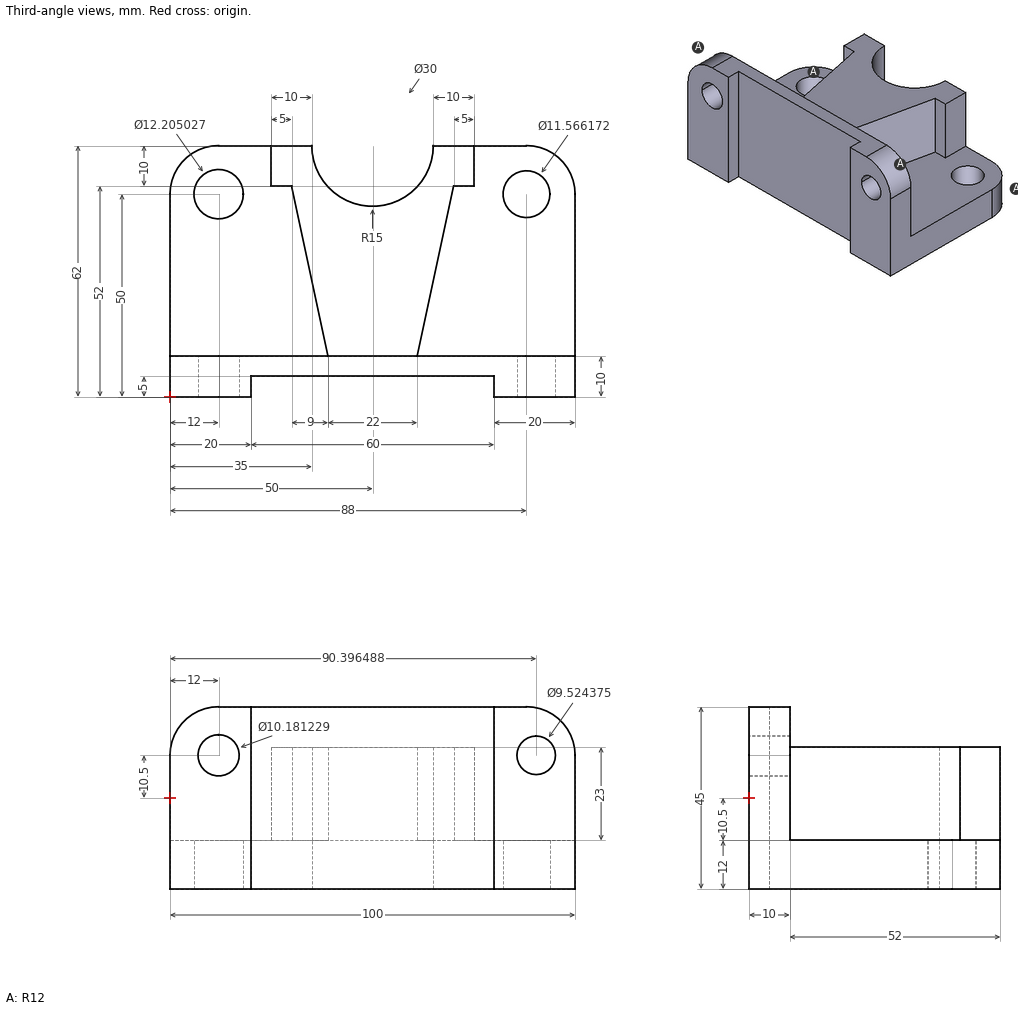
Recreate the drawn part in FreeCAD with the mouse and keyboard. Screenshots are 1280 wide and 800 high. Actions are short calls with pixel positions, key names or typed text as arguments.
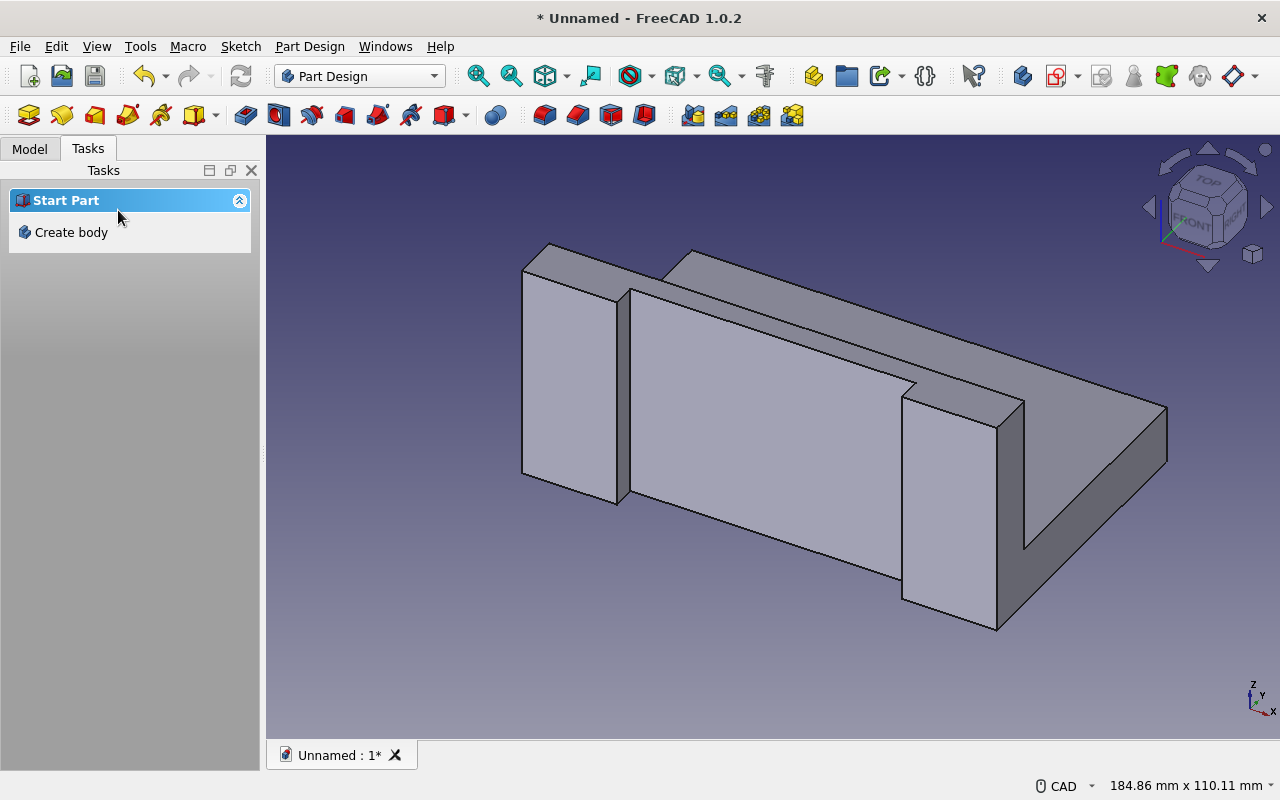
key(v)
key(f)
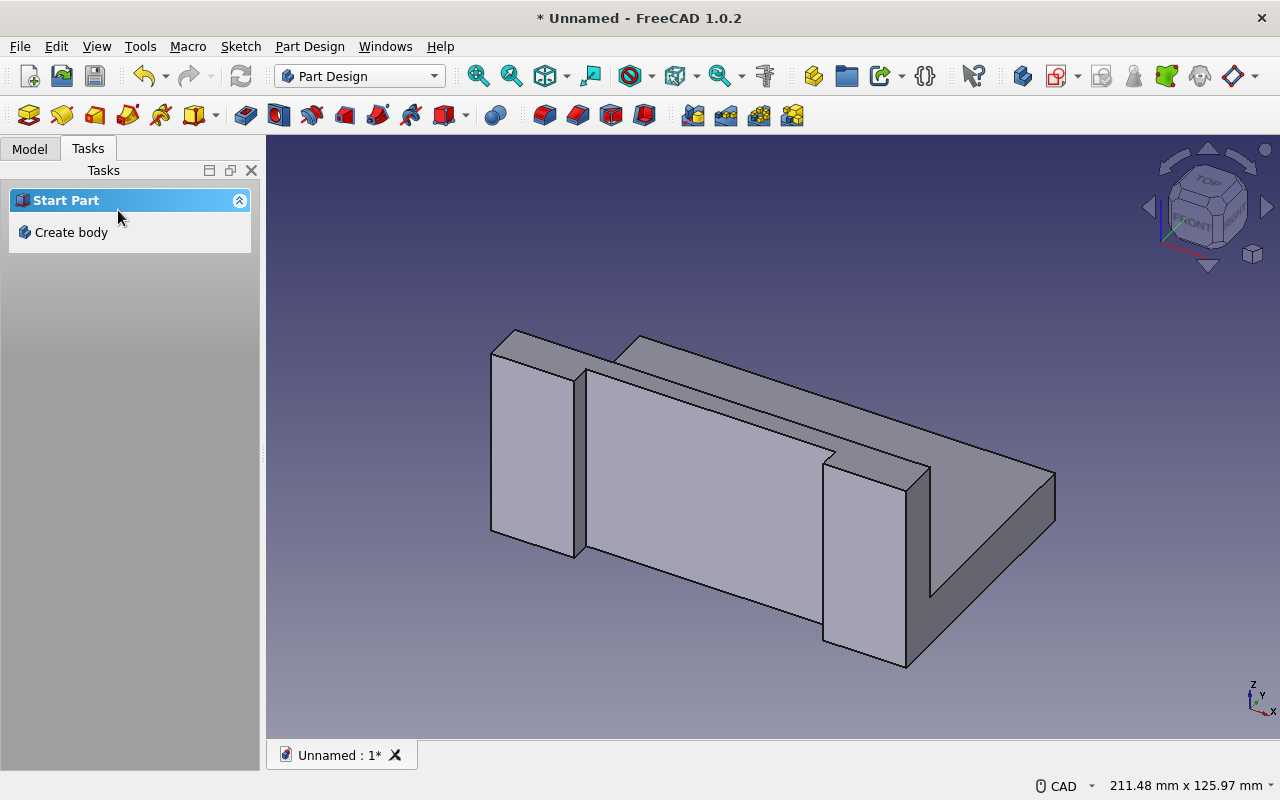
key(0)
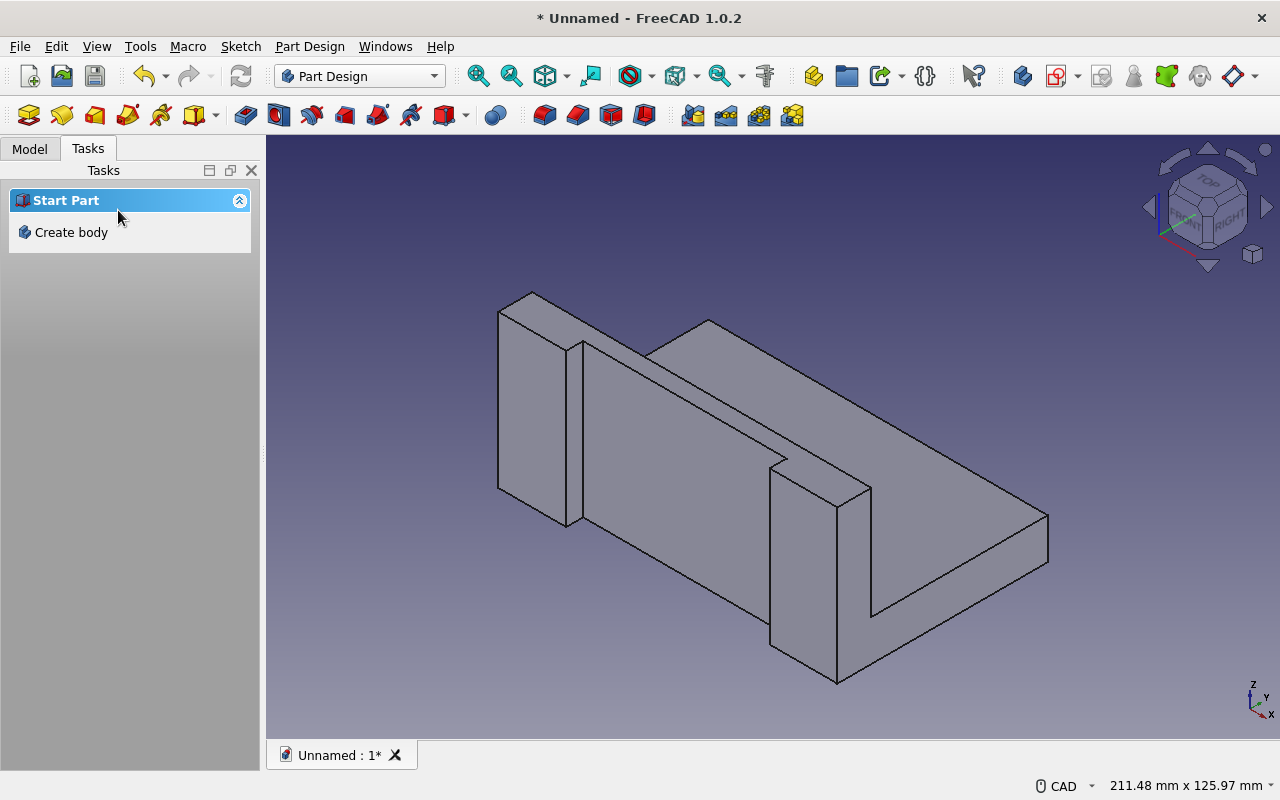
click(887, 523)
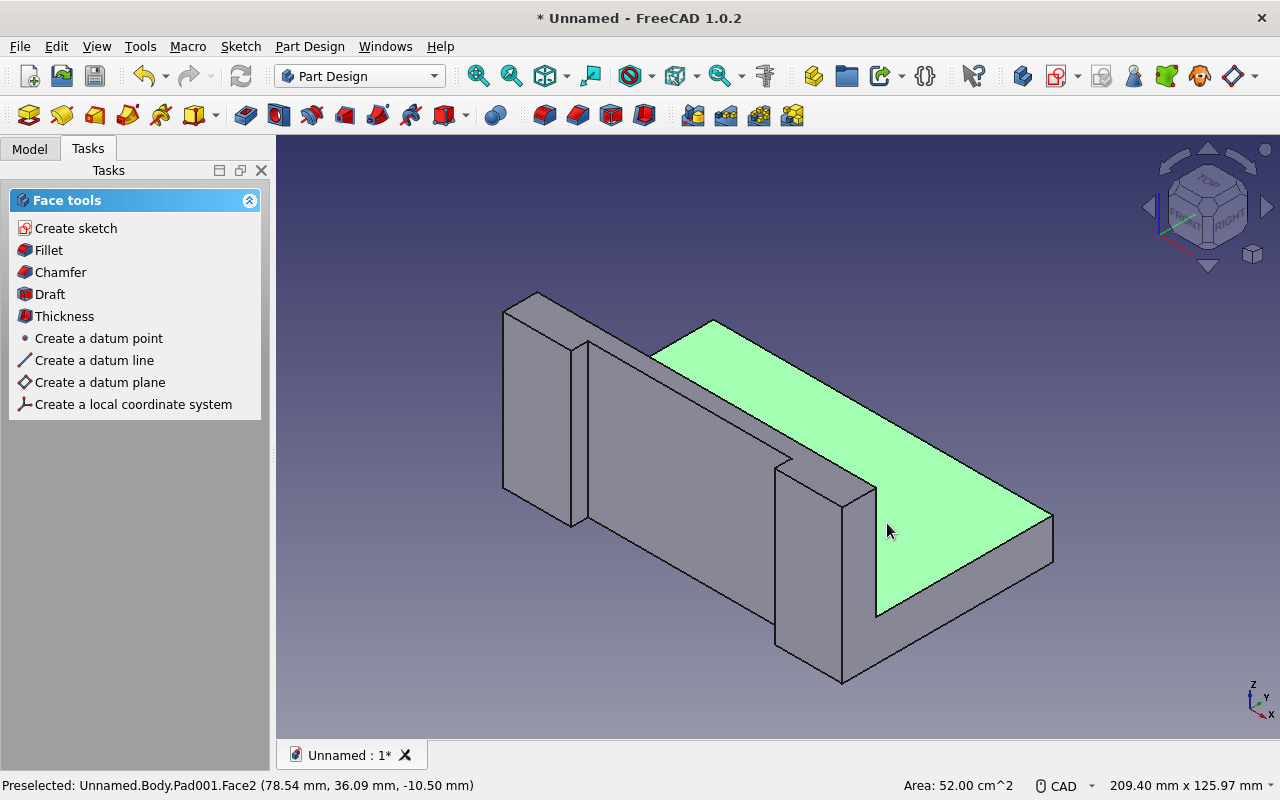
click(1056, 76)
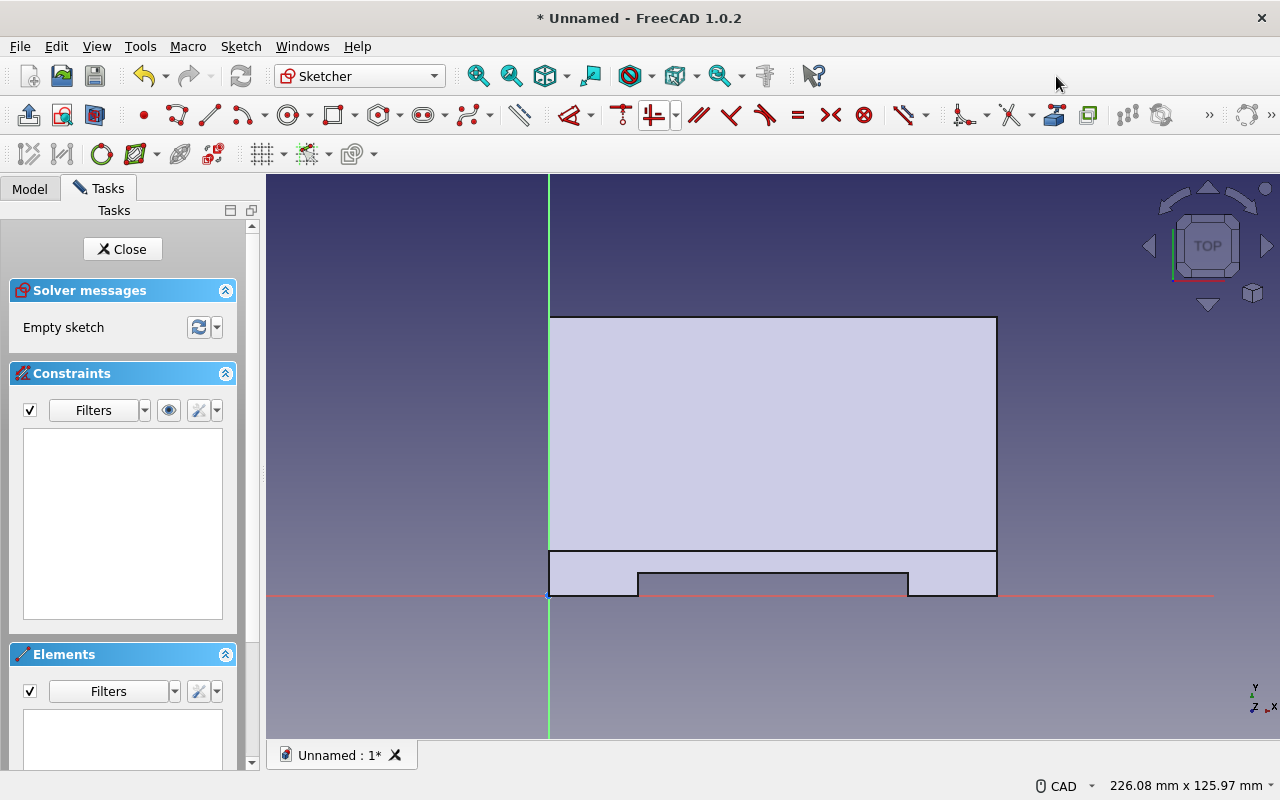
click(95, 116)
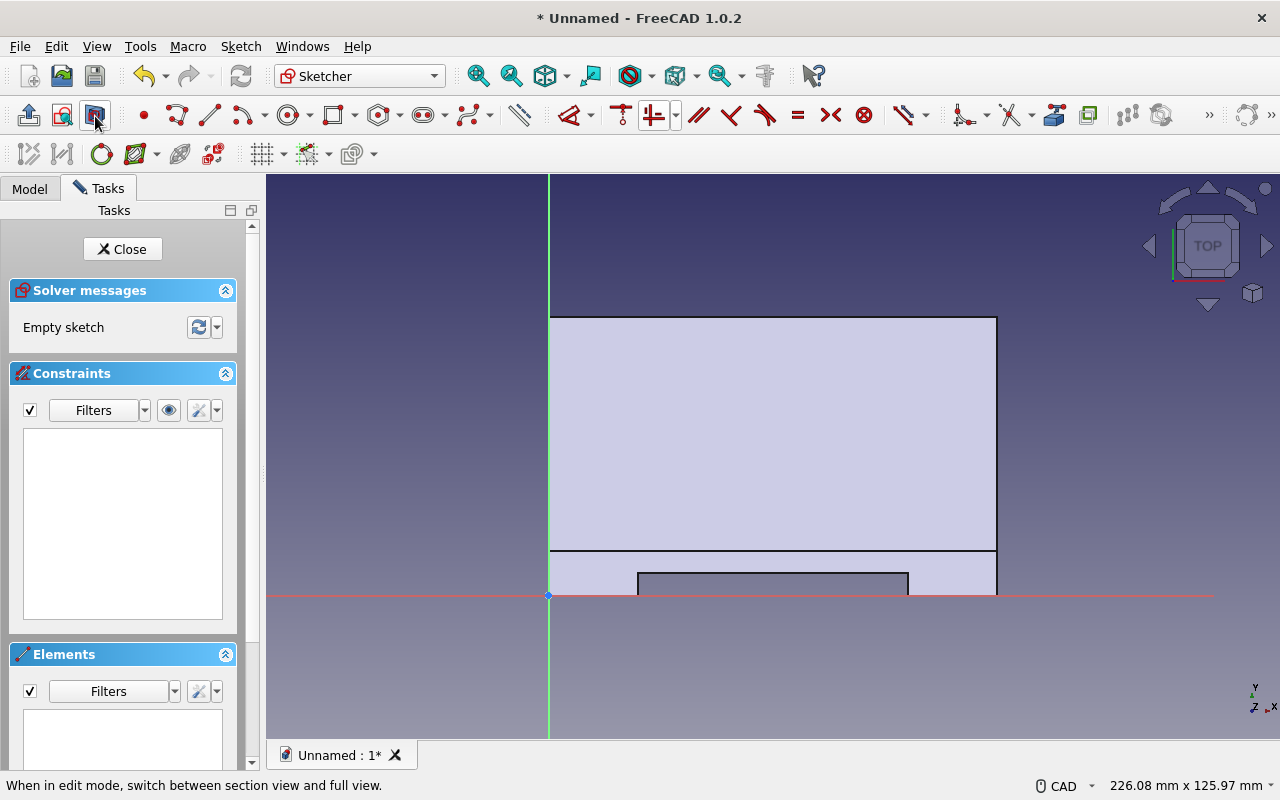
key(g)
key(m)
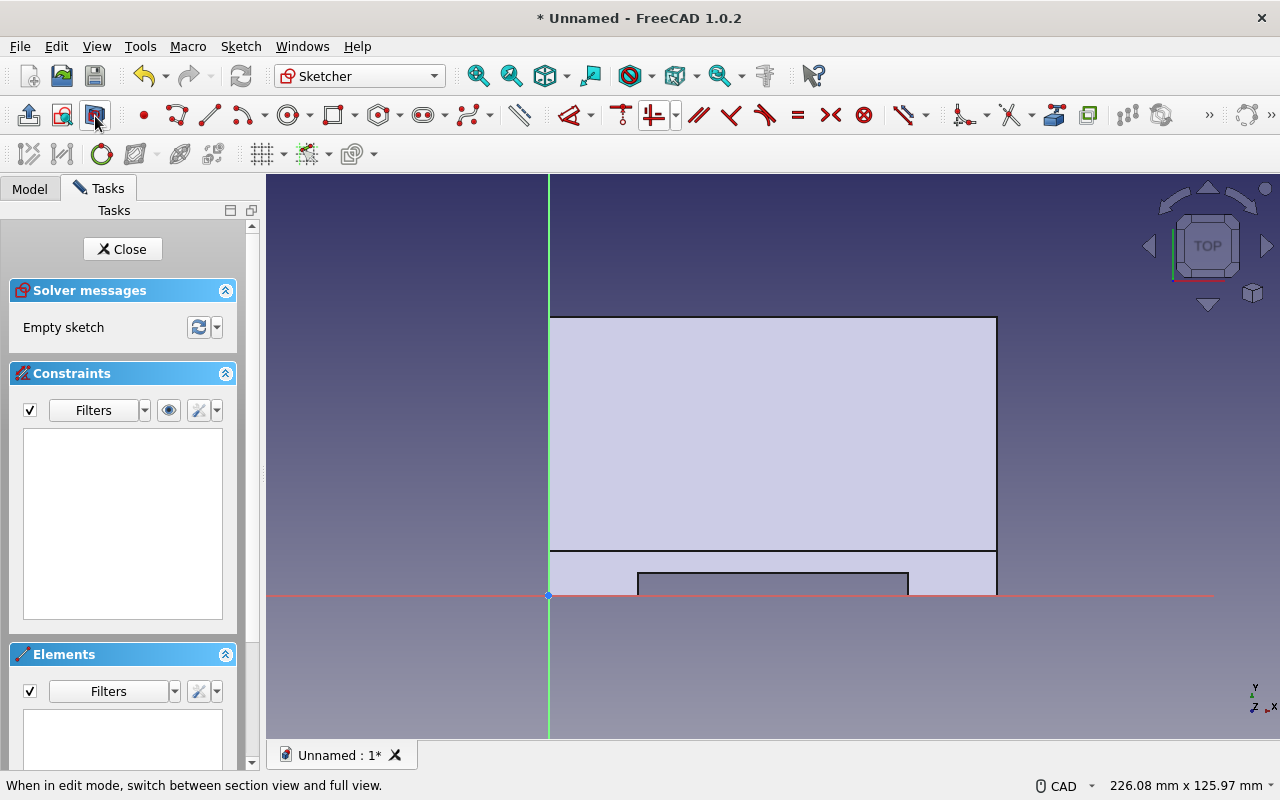
click(706, 317)
click(661, 317)
click(661, 362)
click(683, 362)
click(724, 551)
click(822, 551)
click(863, 362)
click(885, 362)
click(885, 317)
click(840, 317)
right_click(840, 317)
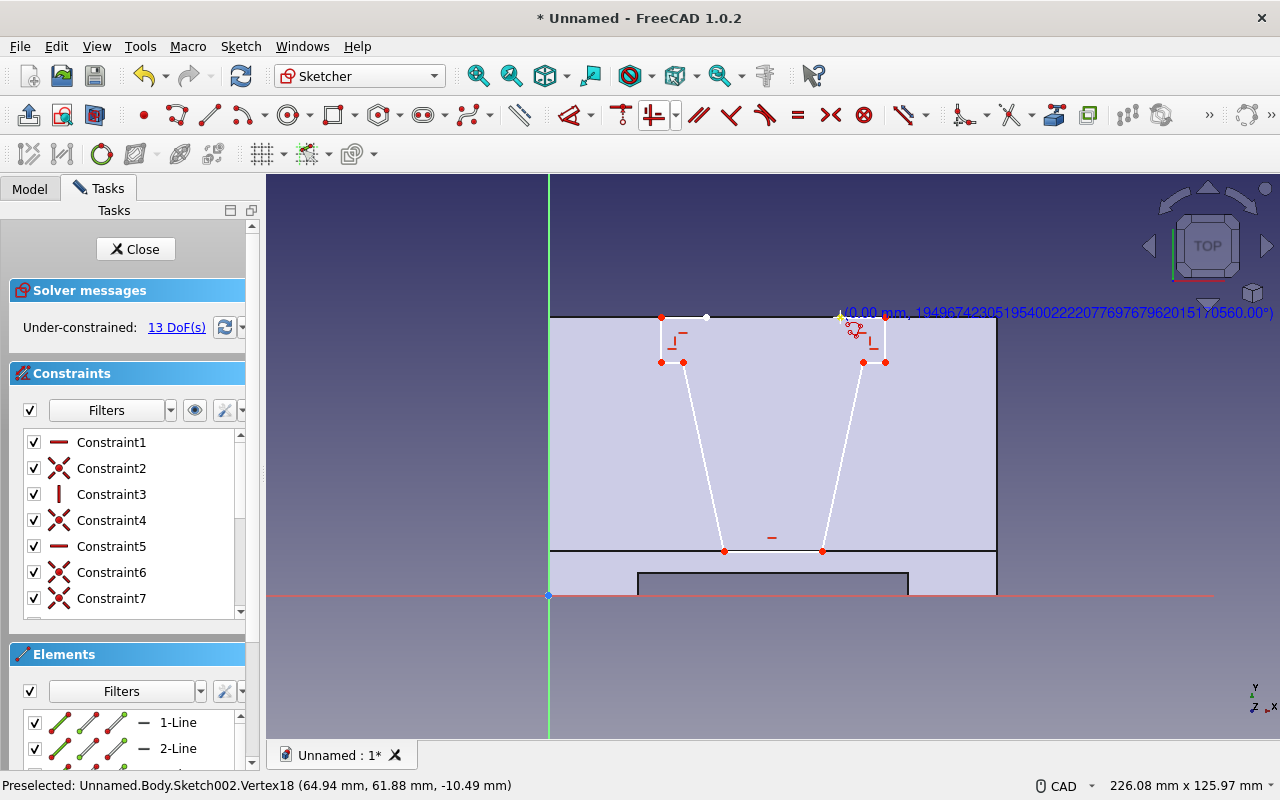
key(g)
key(3)
key(a)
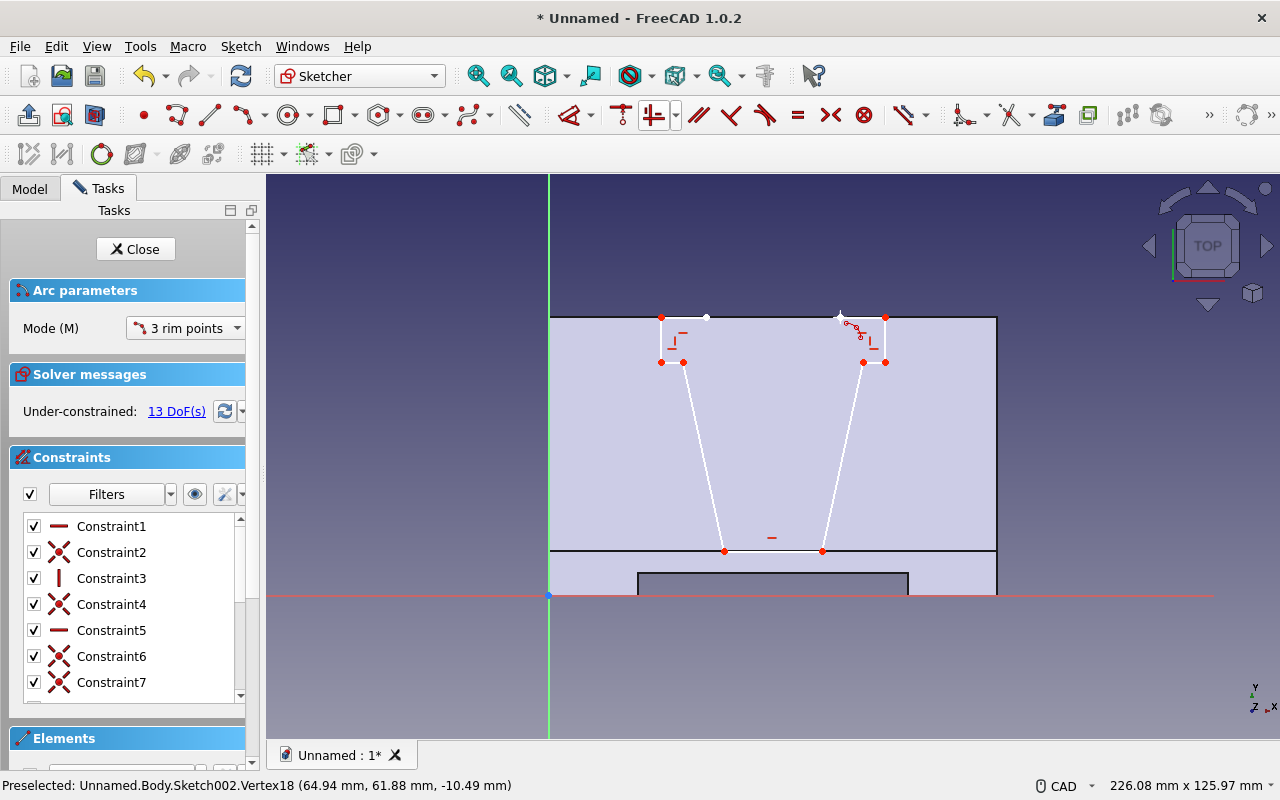
click(840, 318)
click(706, 318)
click(773, 385)
key(Escape)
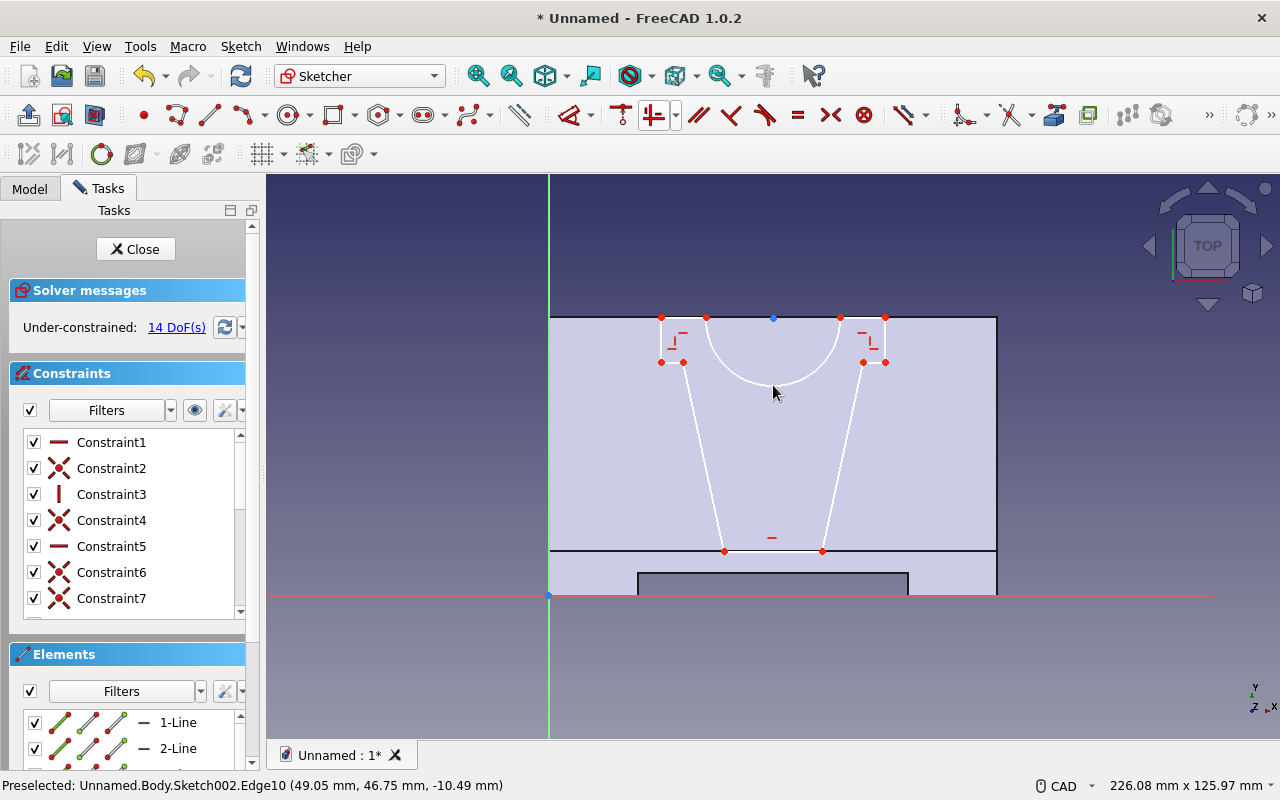
click(733, 373)